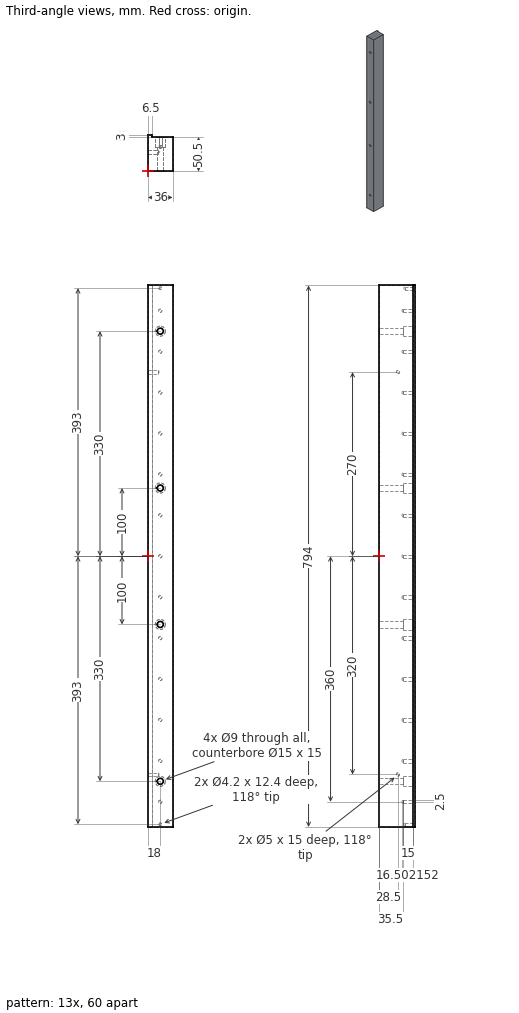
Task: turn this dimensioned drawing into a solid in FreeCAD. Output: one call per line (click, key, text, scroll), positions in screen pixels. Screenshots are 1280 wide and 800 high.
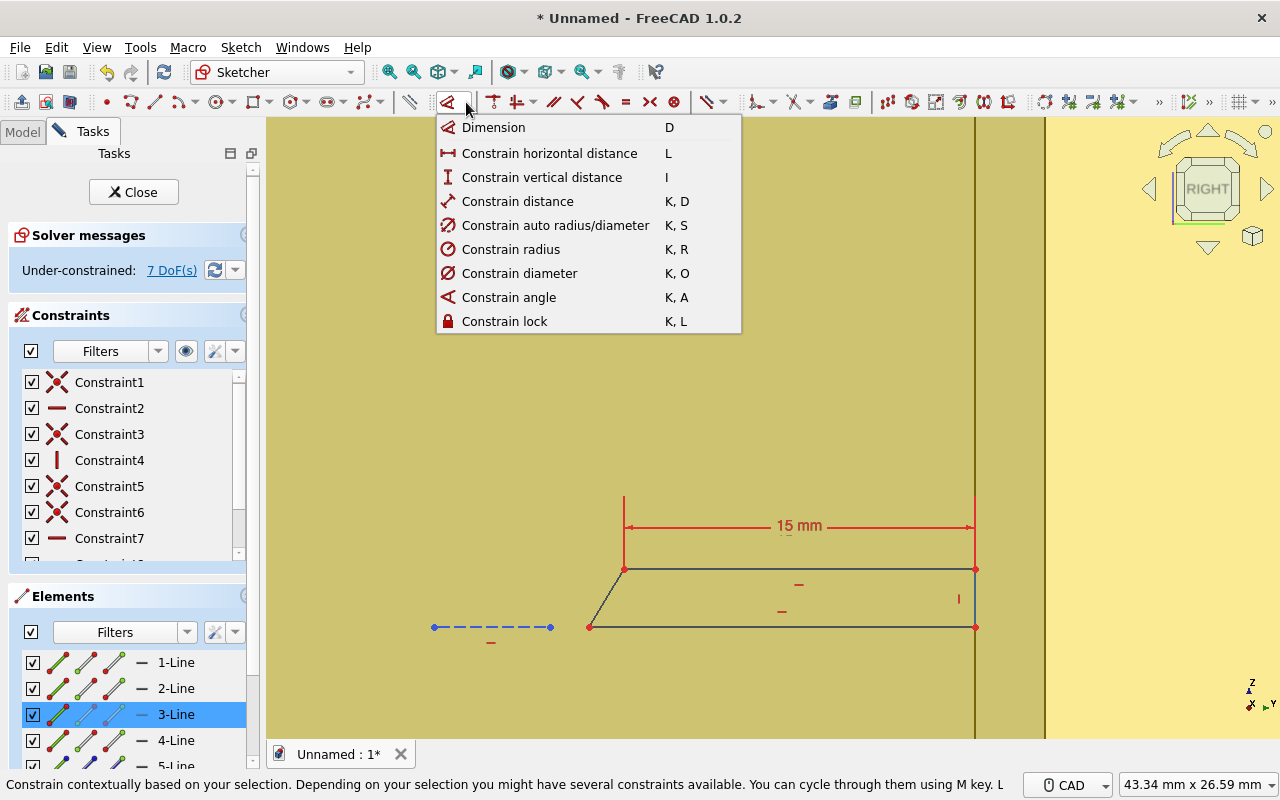
click(589, 177)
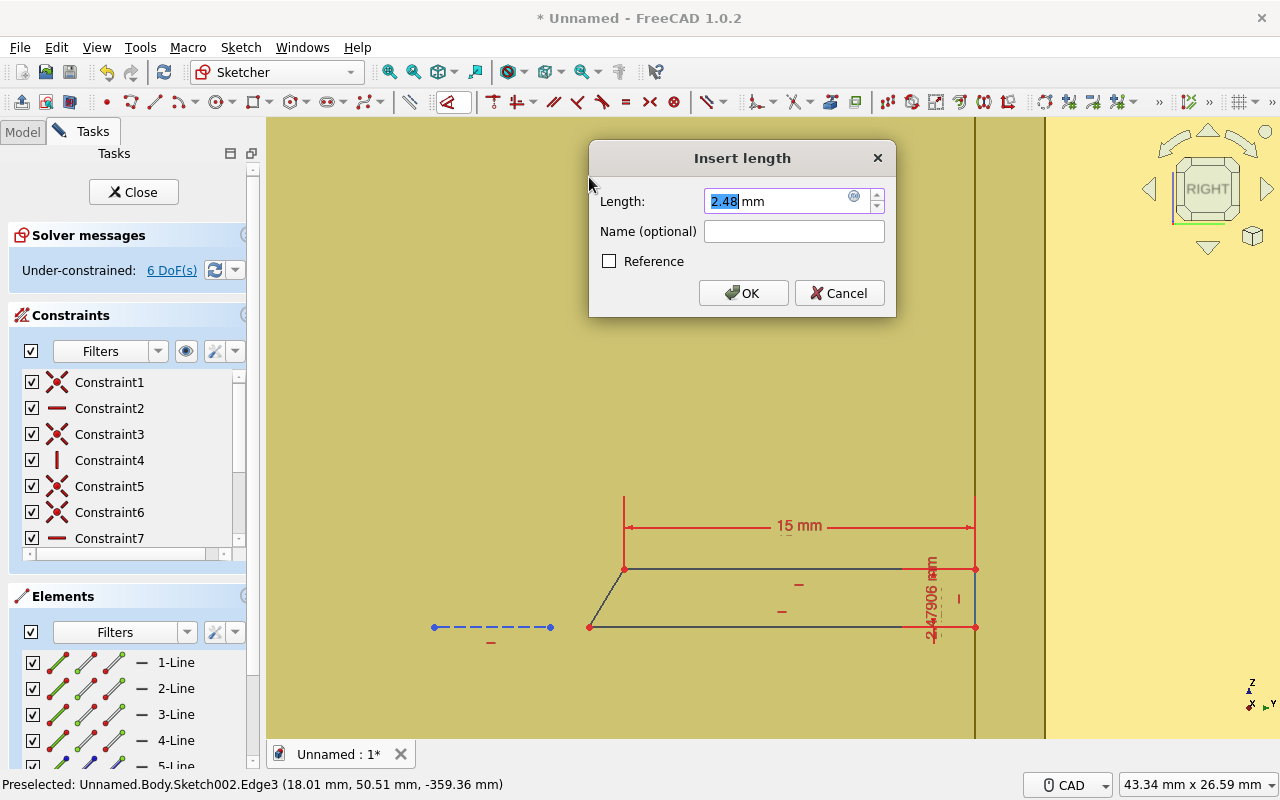
text(2.5)
key(Return)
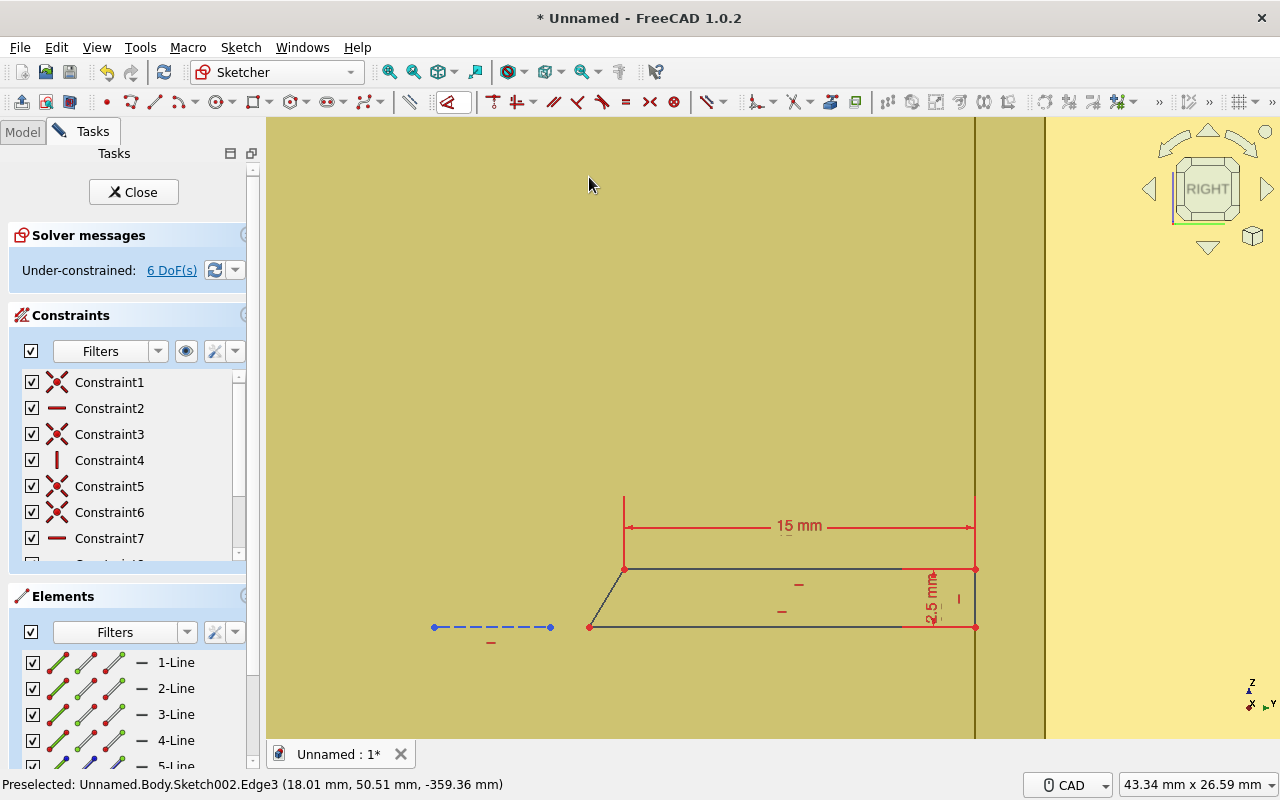
click(589, 627)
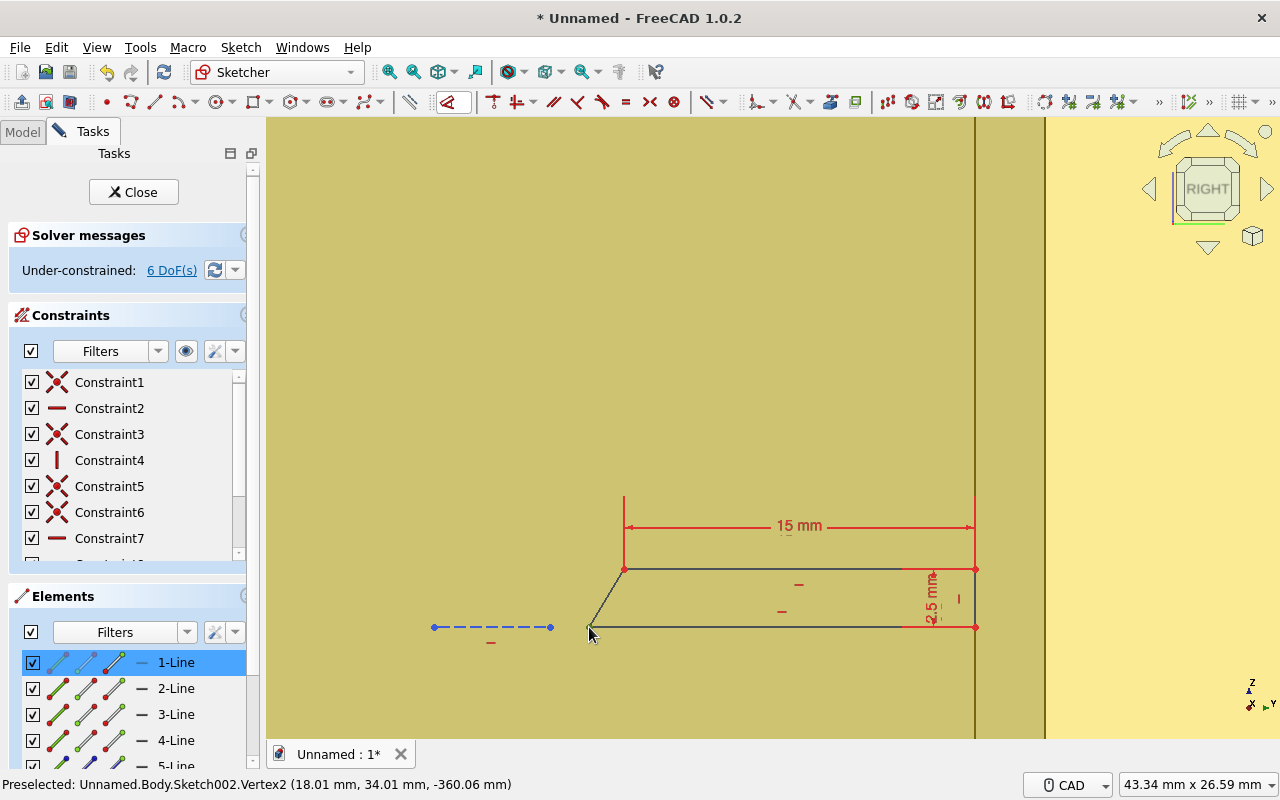
click(466, 102)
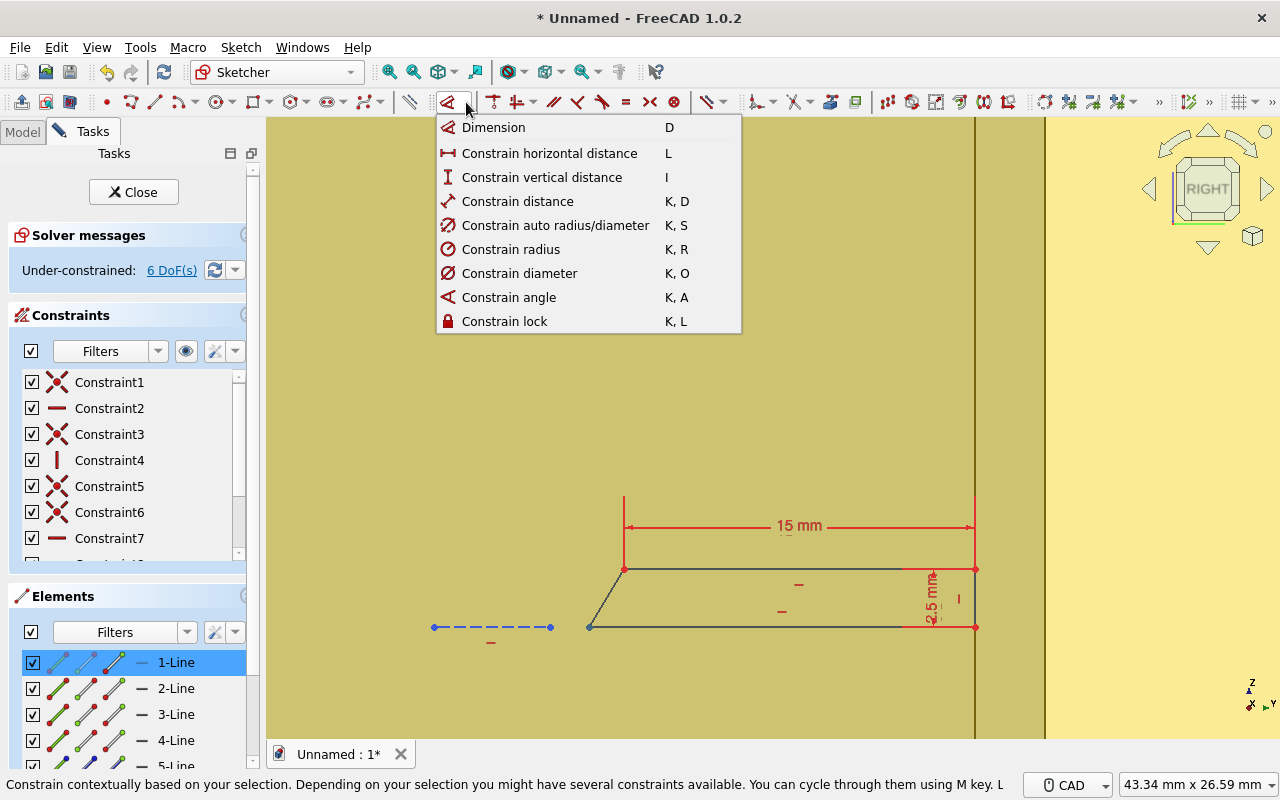
click(589, 177)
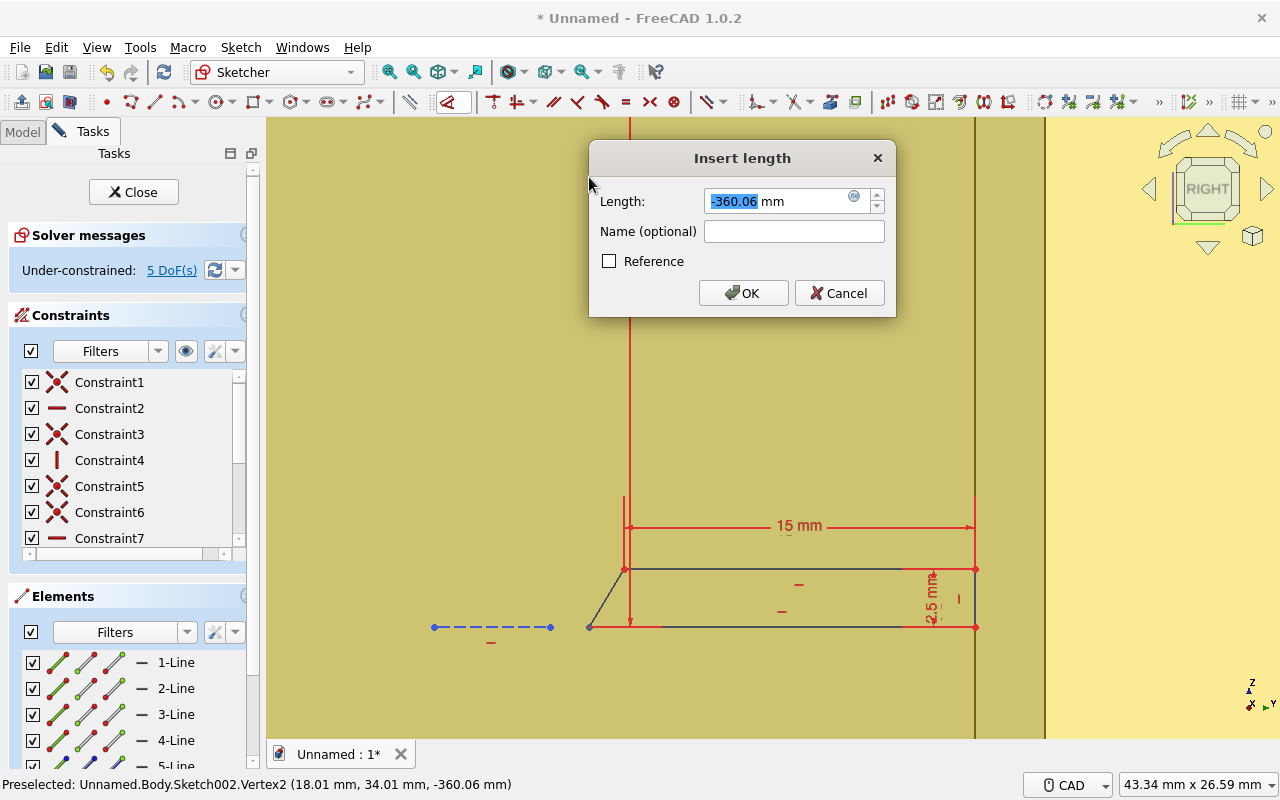
text(-360)
key(Return)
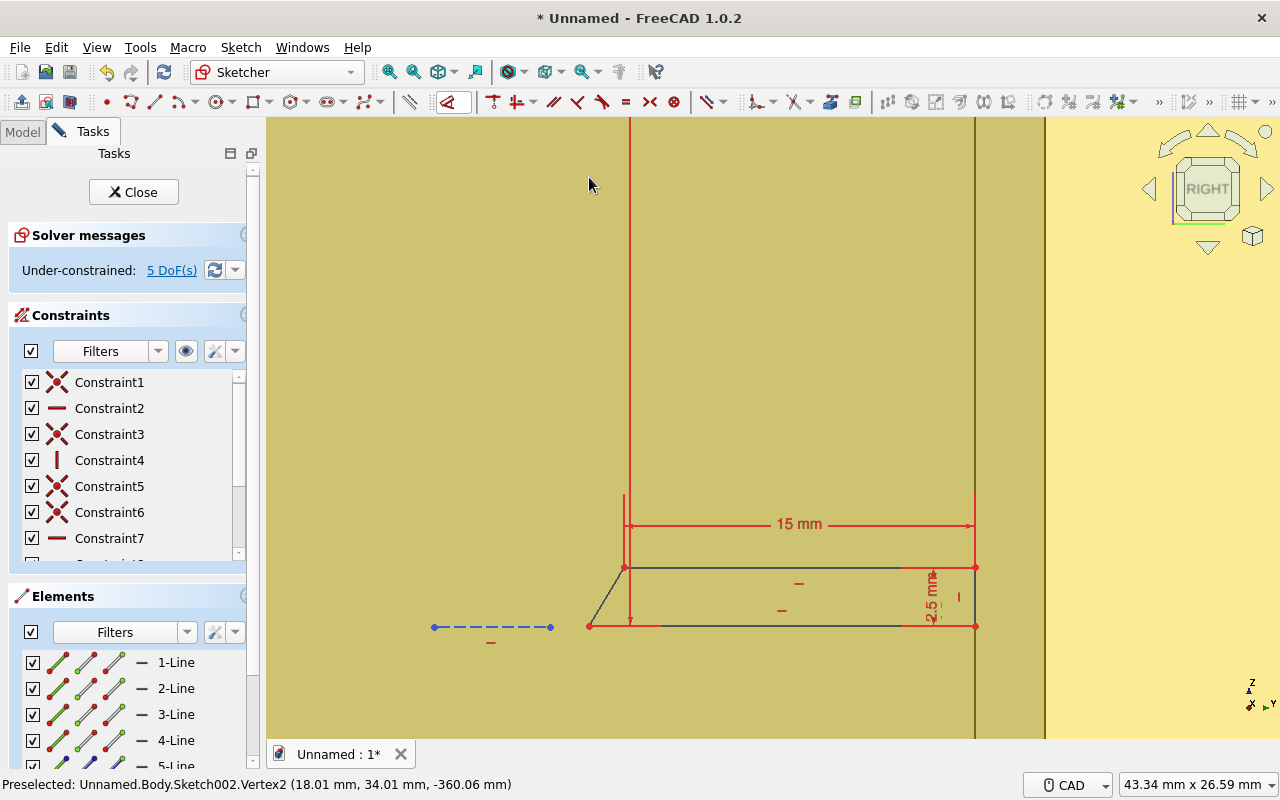
click(550, 627)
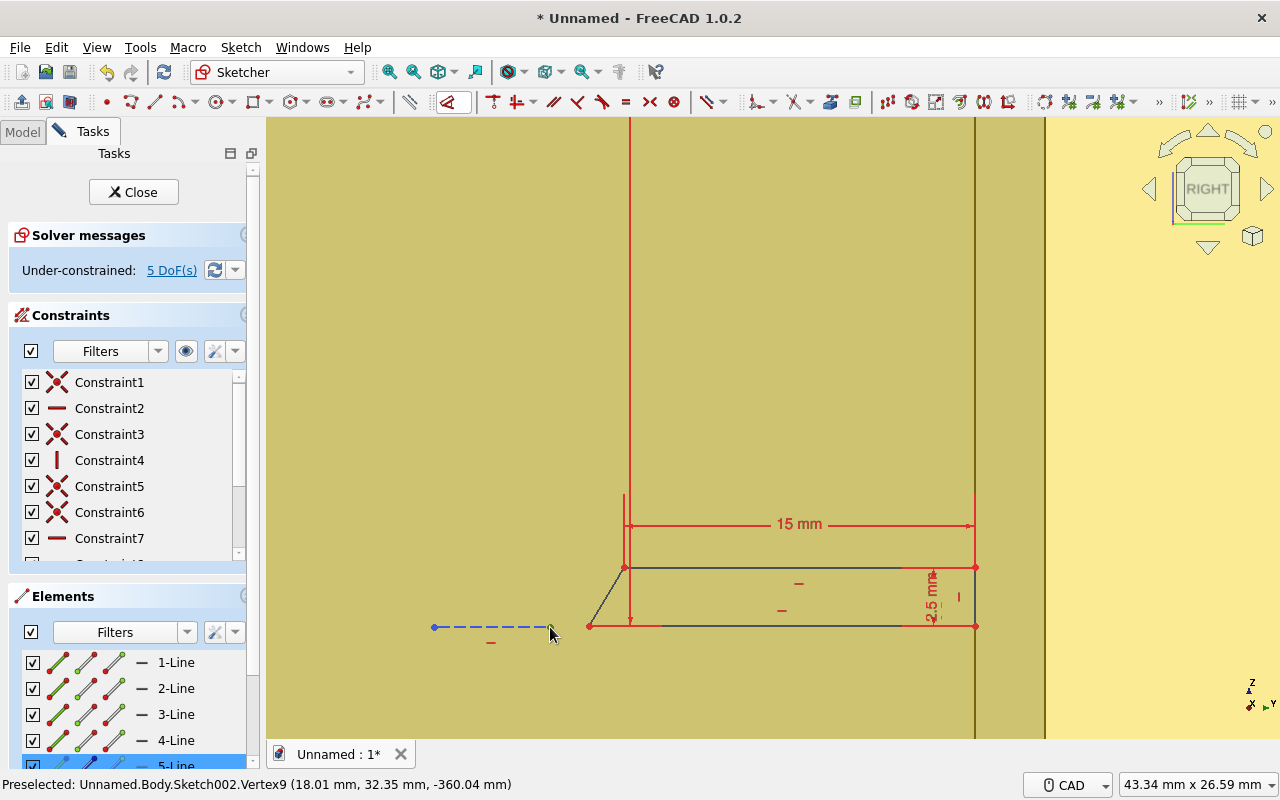
click(466, 102)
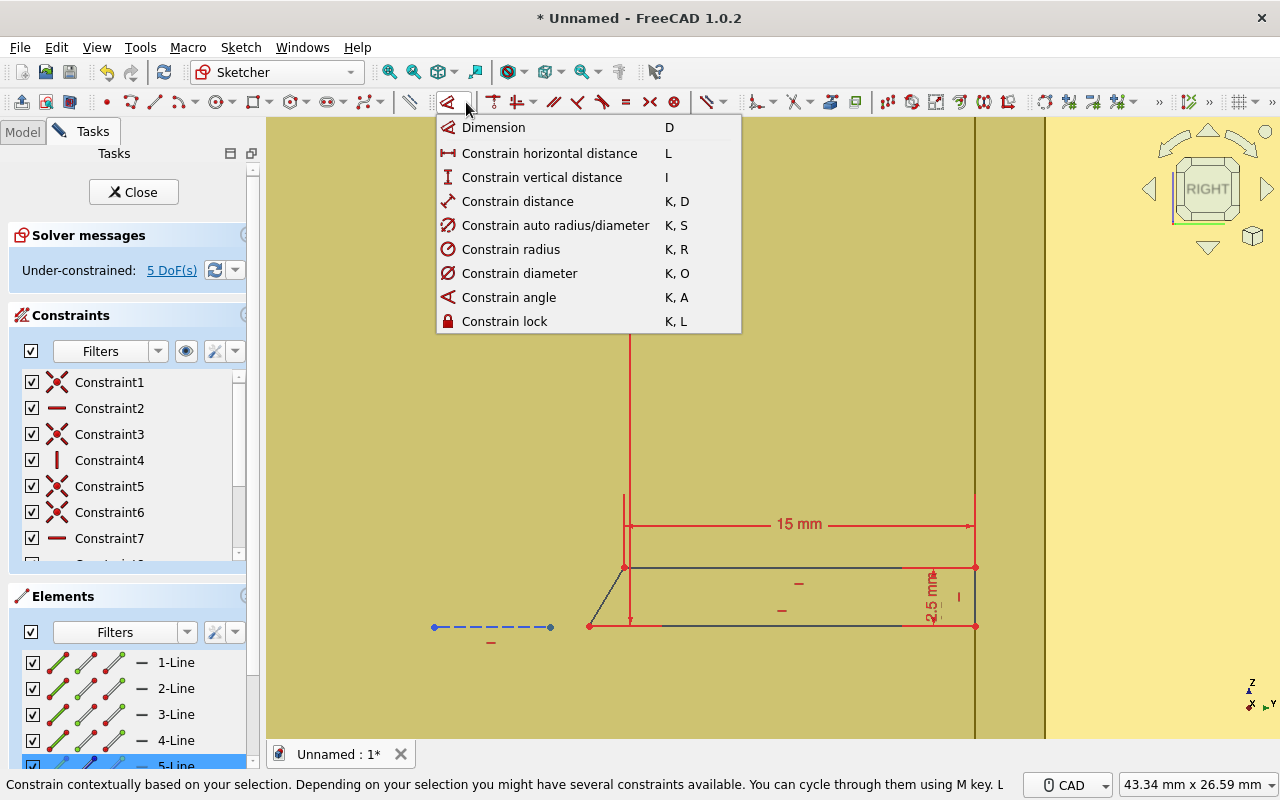
click(589, 177)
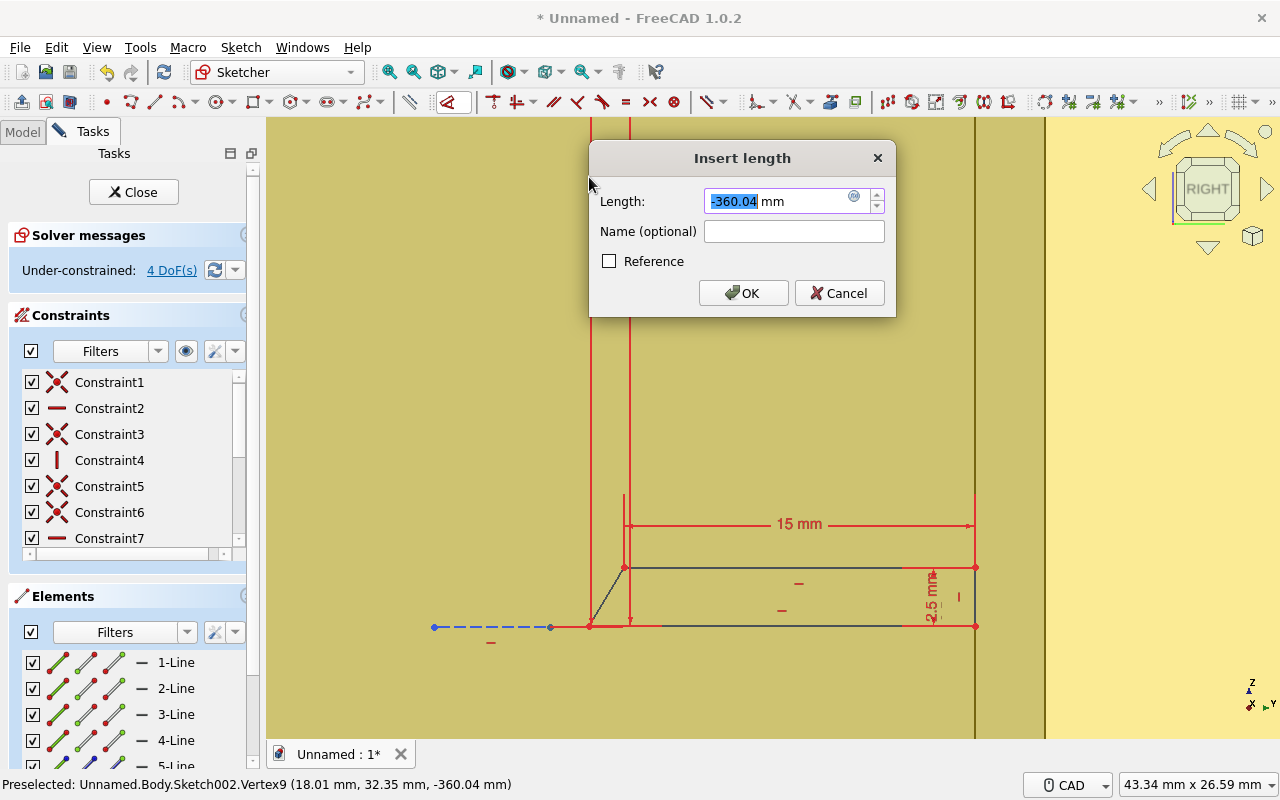
text(-360)
key(Return)